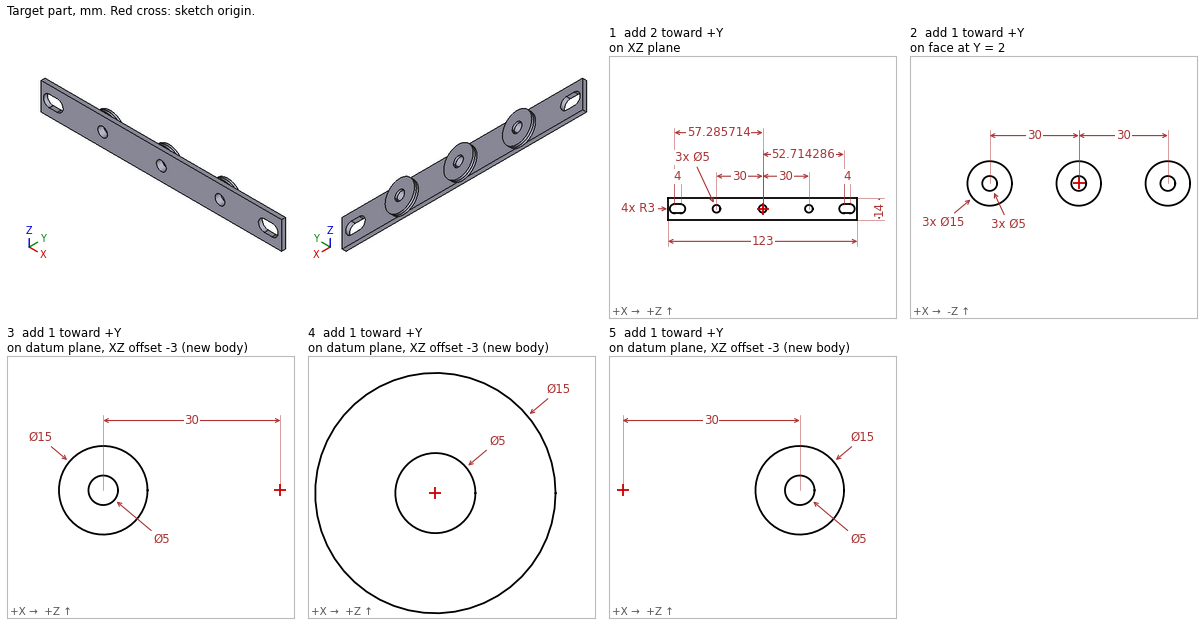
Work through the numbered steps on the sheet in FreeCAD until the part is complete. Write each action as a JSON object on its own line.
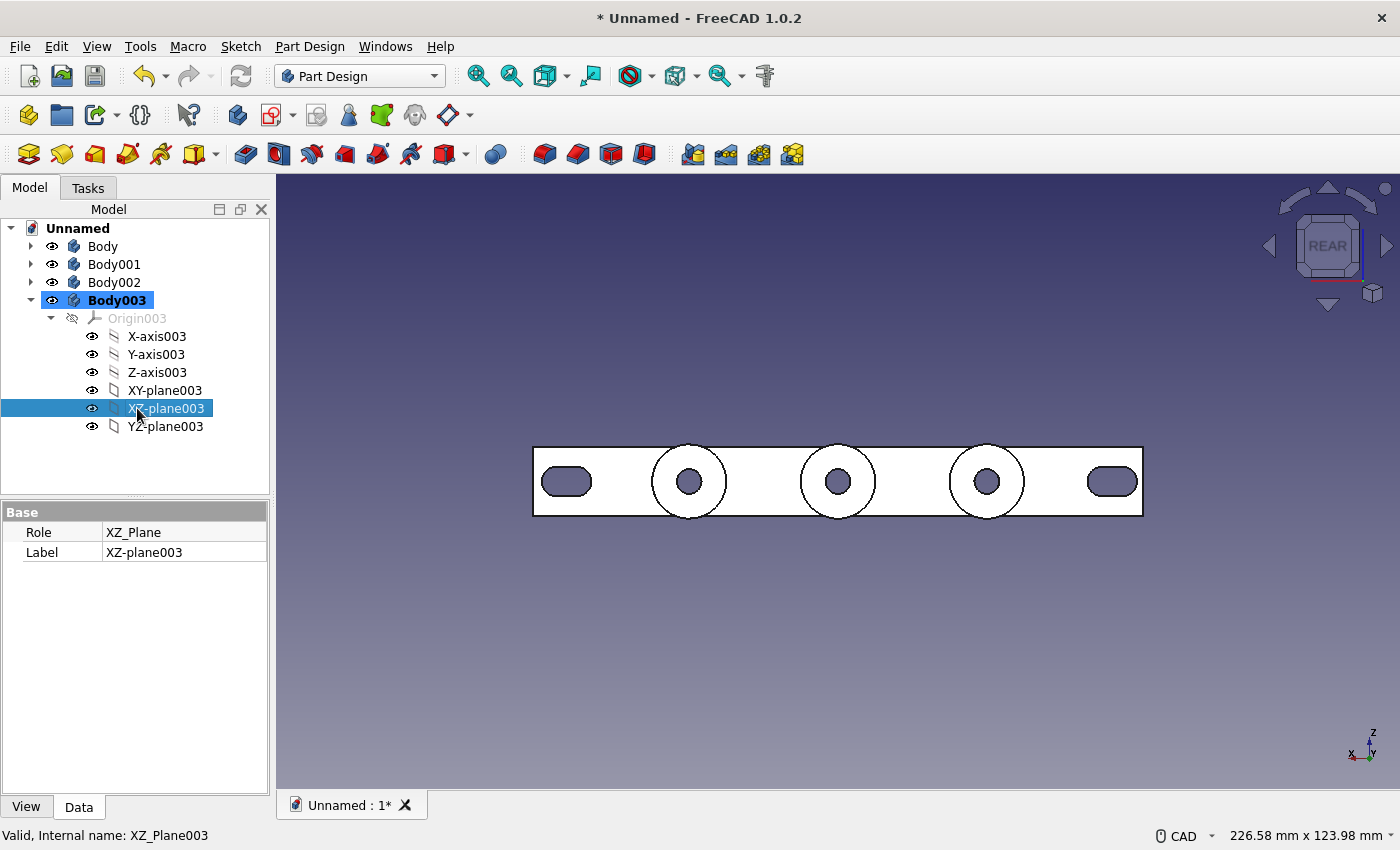
{"action": "left_click", "coordinate": [448, 116]}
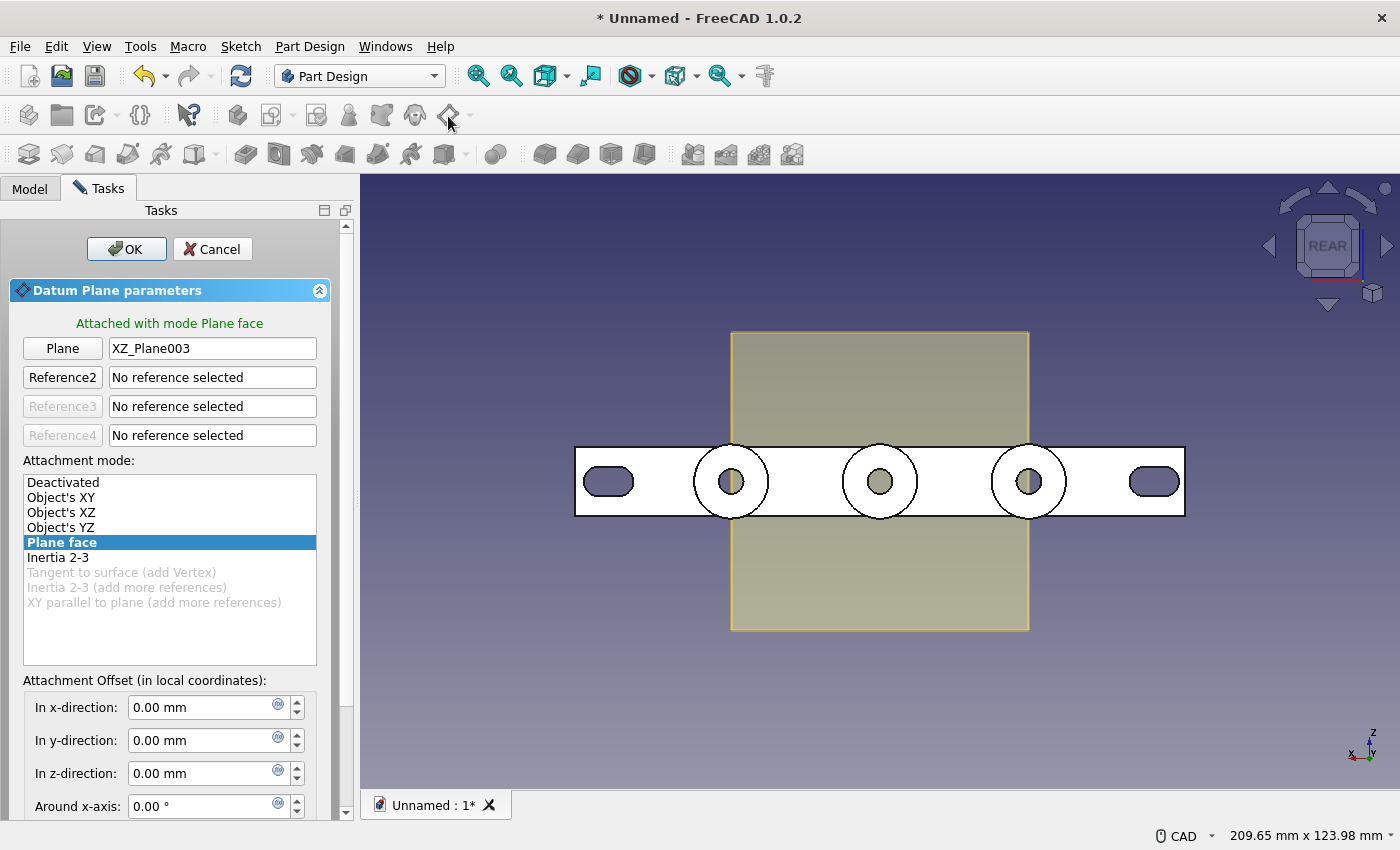
{"action": "triple_click", "coordinate": [210, 774]}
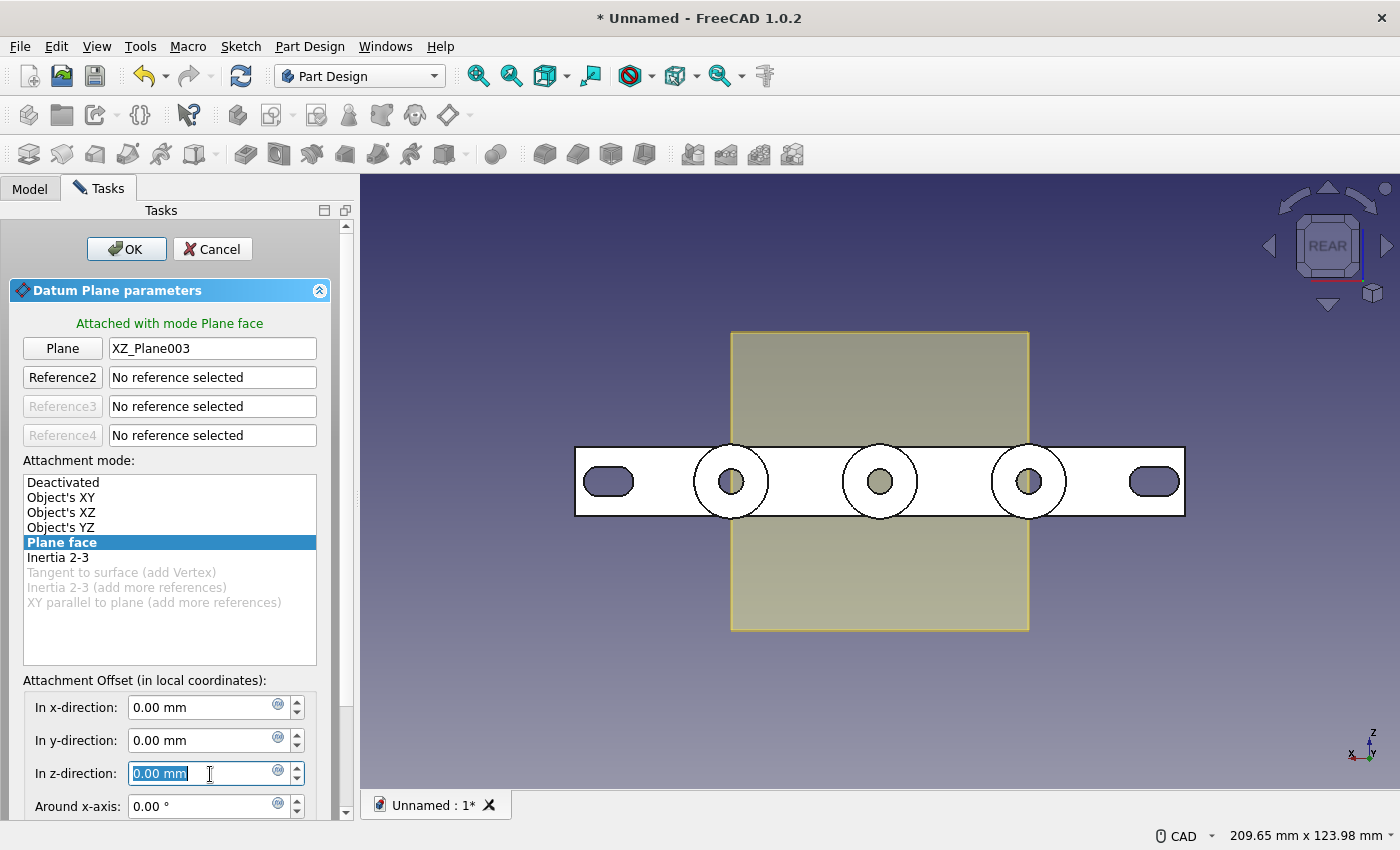
{"action": "type", "text": "-3"}
{"action": "key", "text": "Tab"}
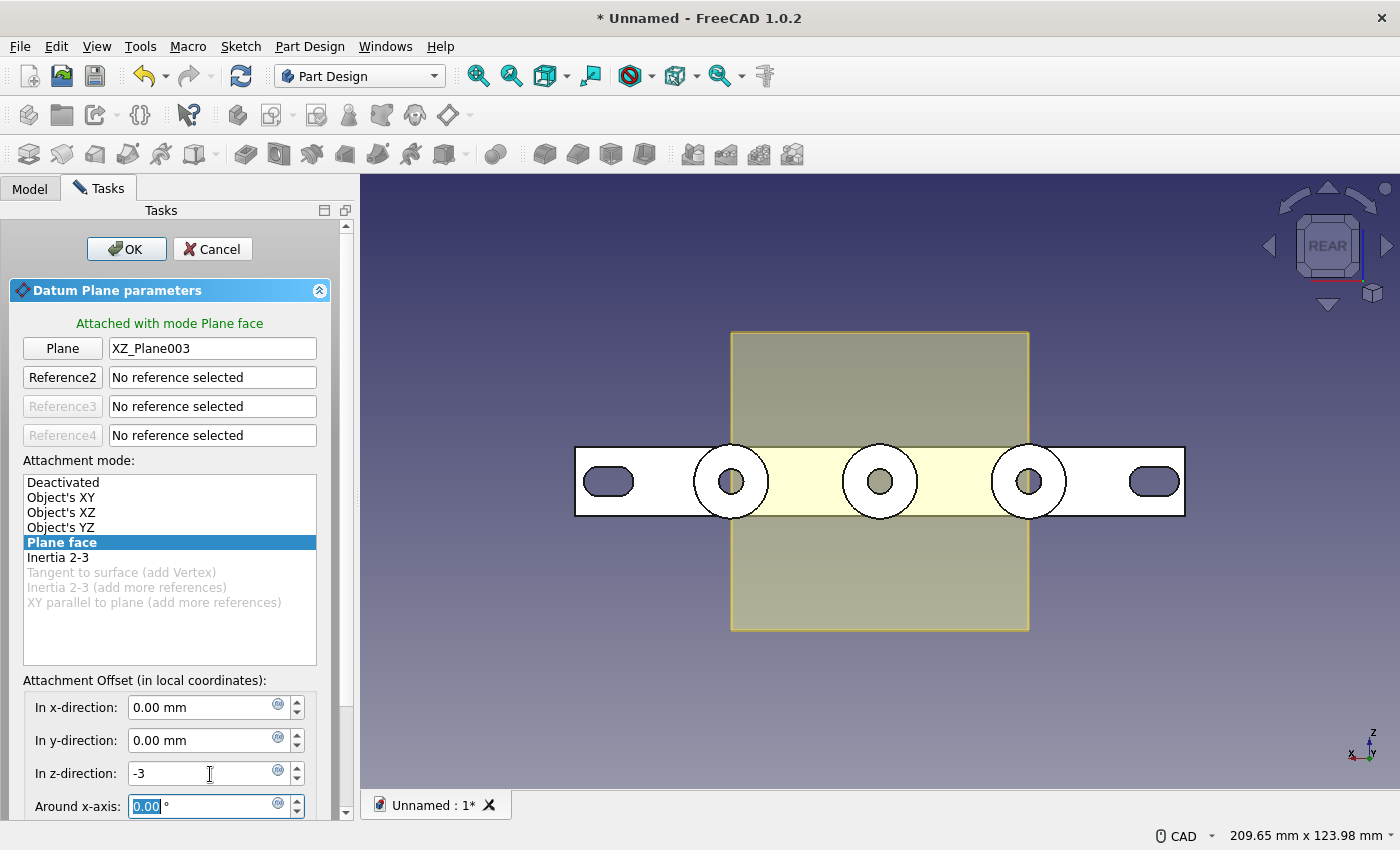
{"action": "left_click", "coordinate": [127, 249]}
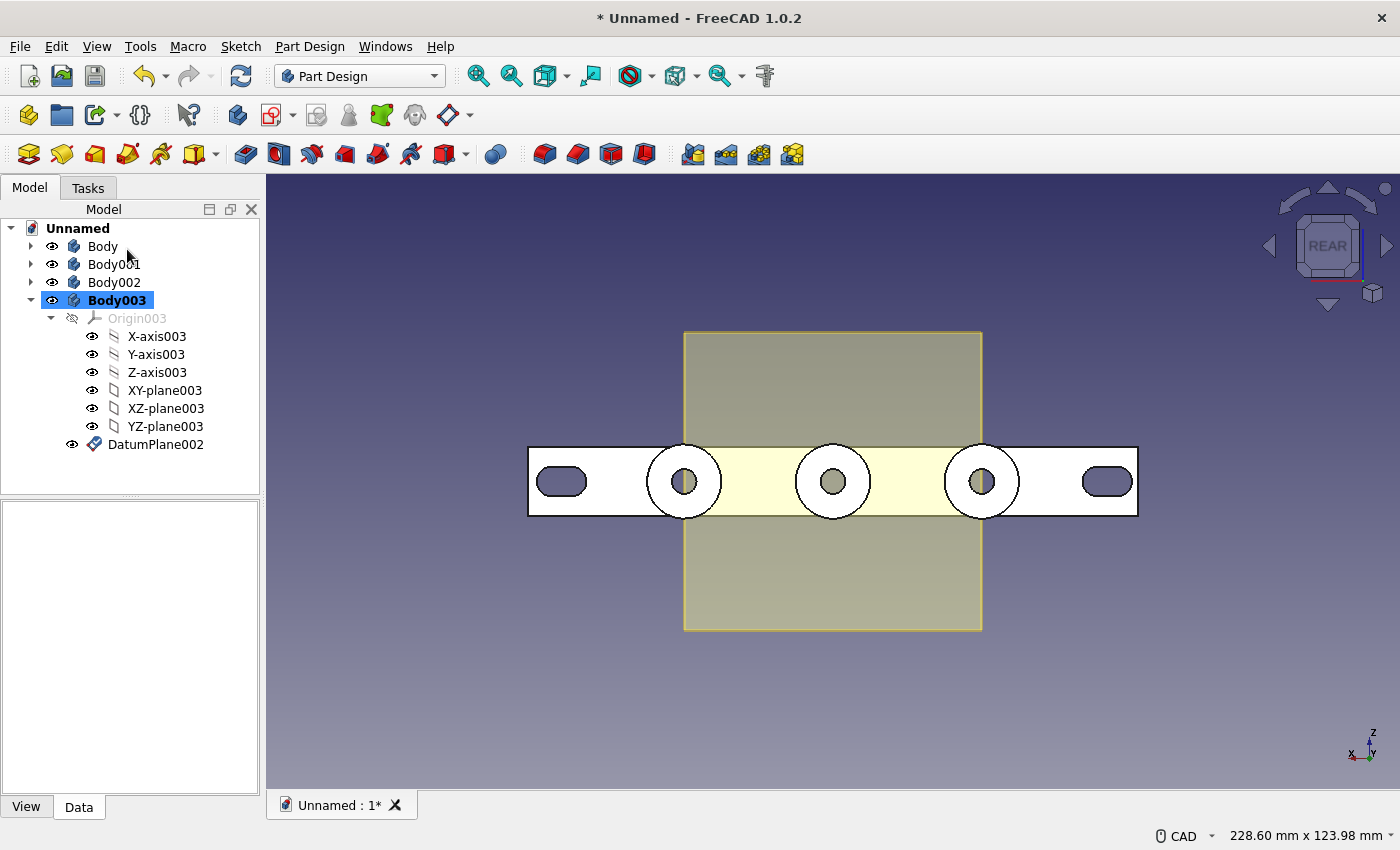
{"action": "left_click", "coordinate": [117, 444]}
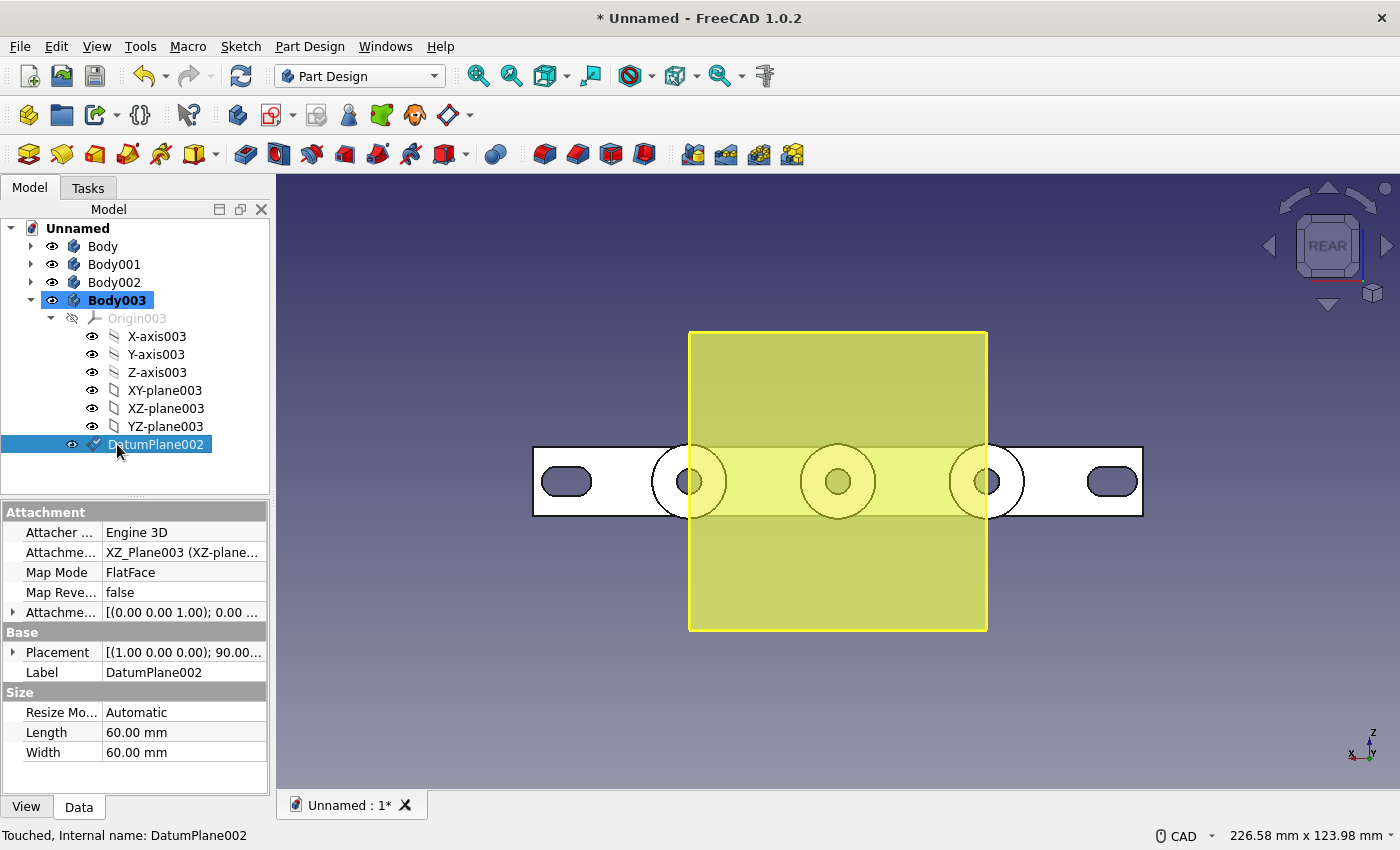
{"action": "left_click", "coordinate": [270, 116]}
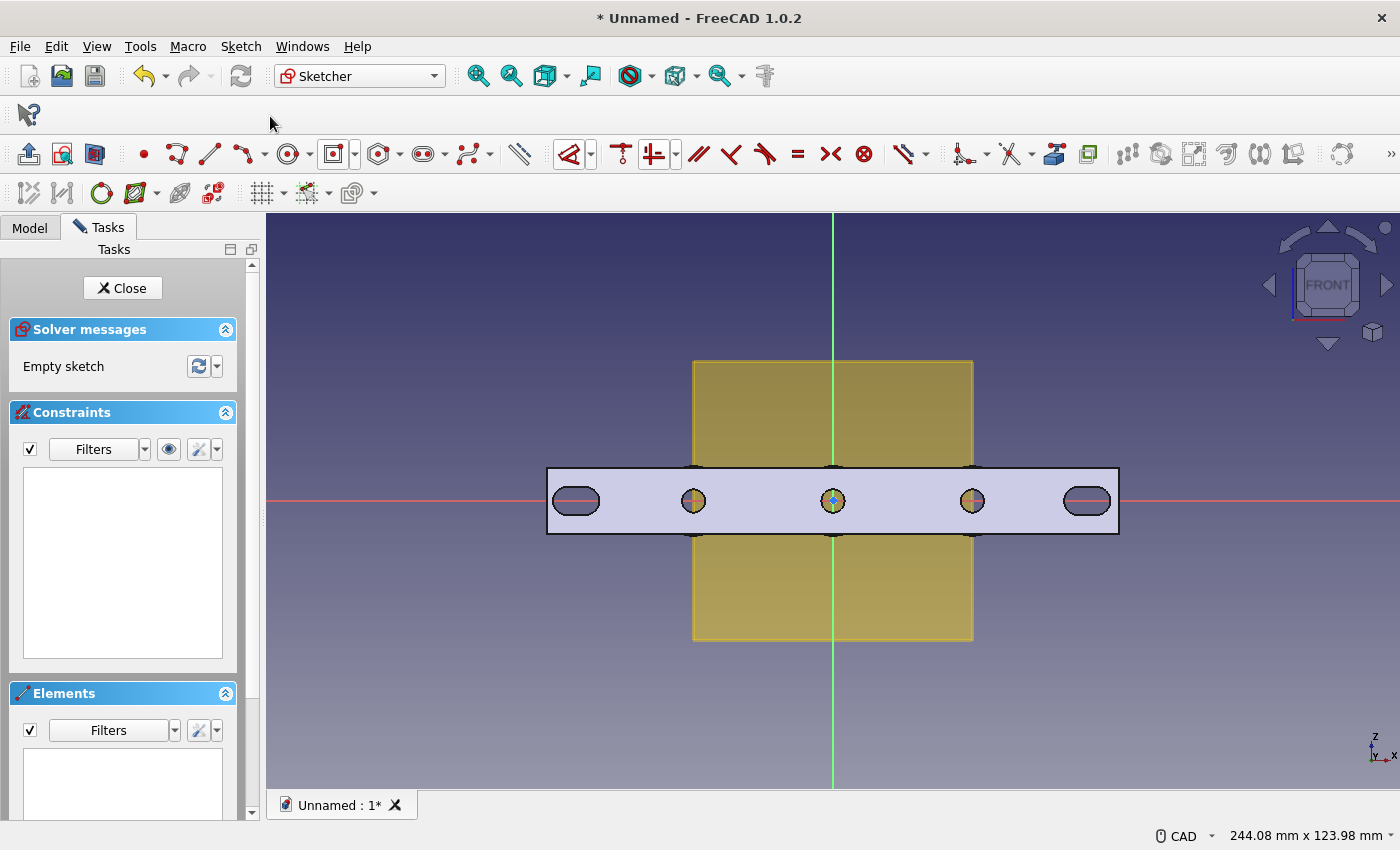
{"action": "scroll", "coordinate": [1025, 501], "scroll_direction": "up", "scroll_amount": 8}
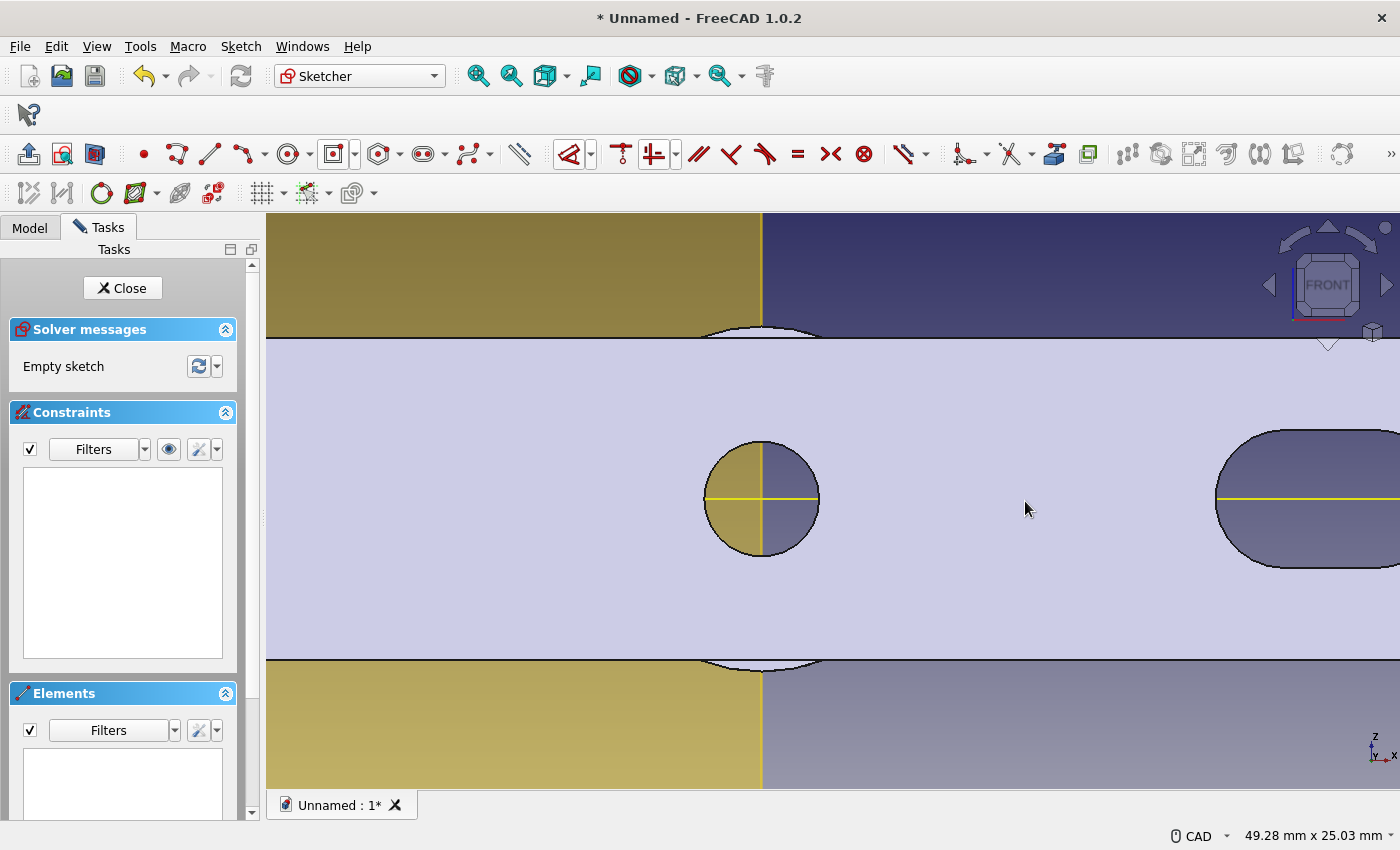
{"action": "left_click", "coordinate": [288, 154]}